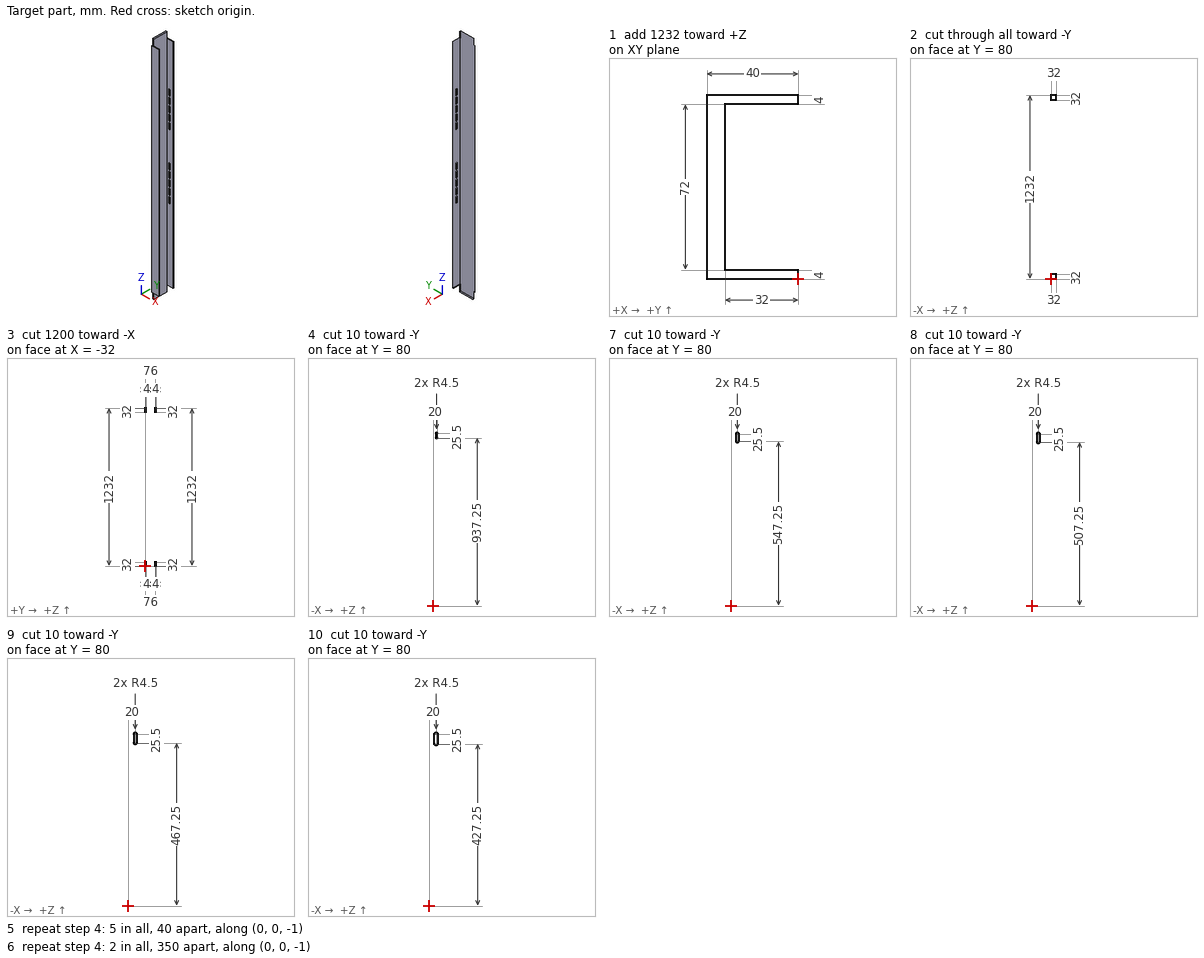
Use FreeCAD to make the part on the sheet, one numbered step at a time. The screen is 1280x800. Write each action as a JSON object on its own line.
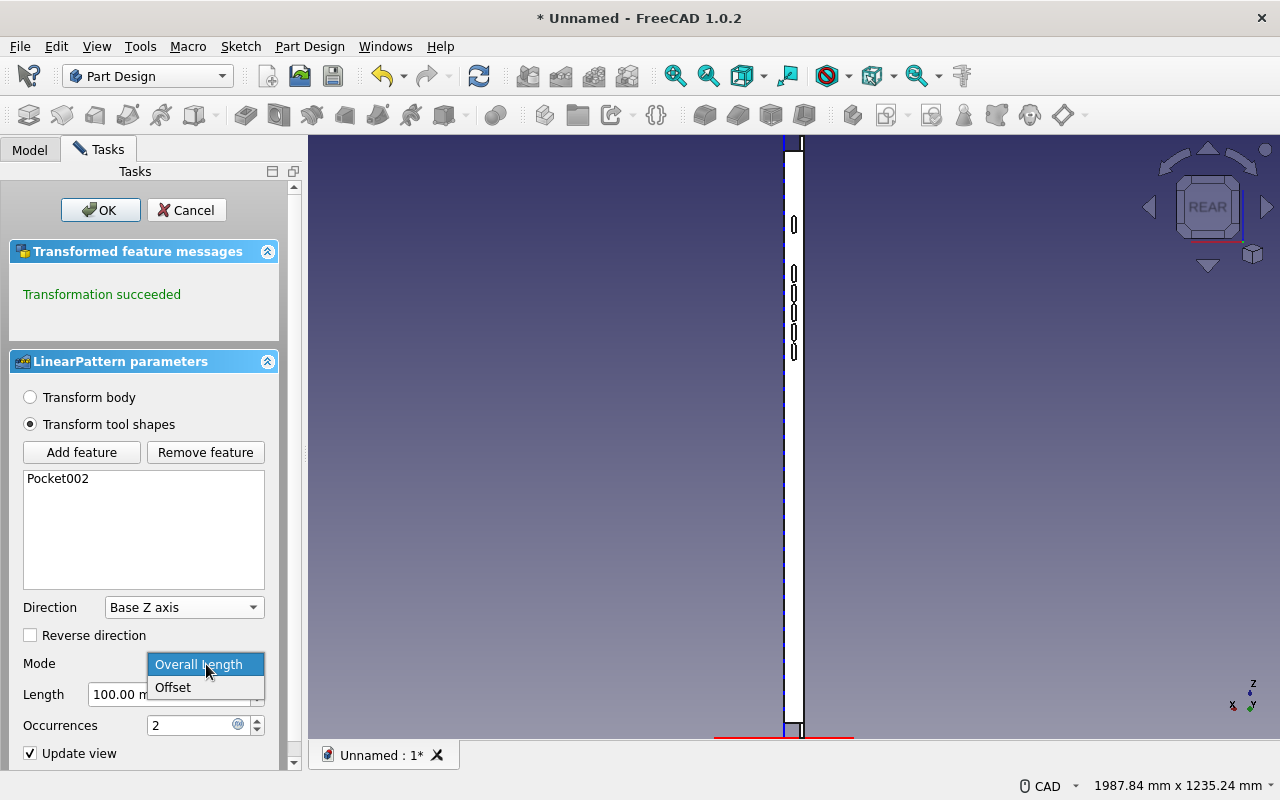
{"action": "left_click", "coordinate": [204, 688]}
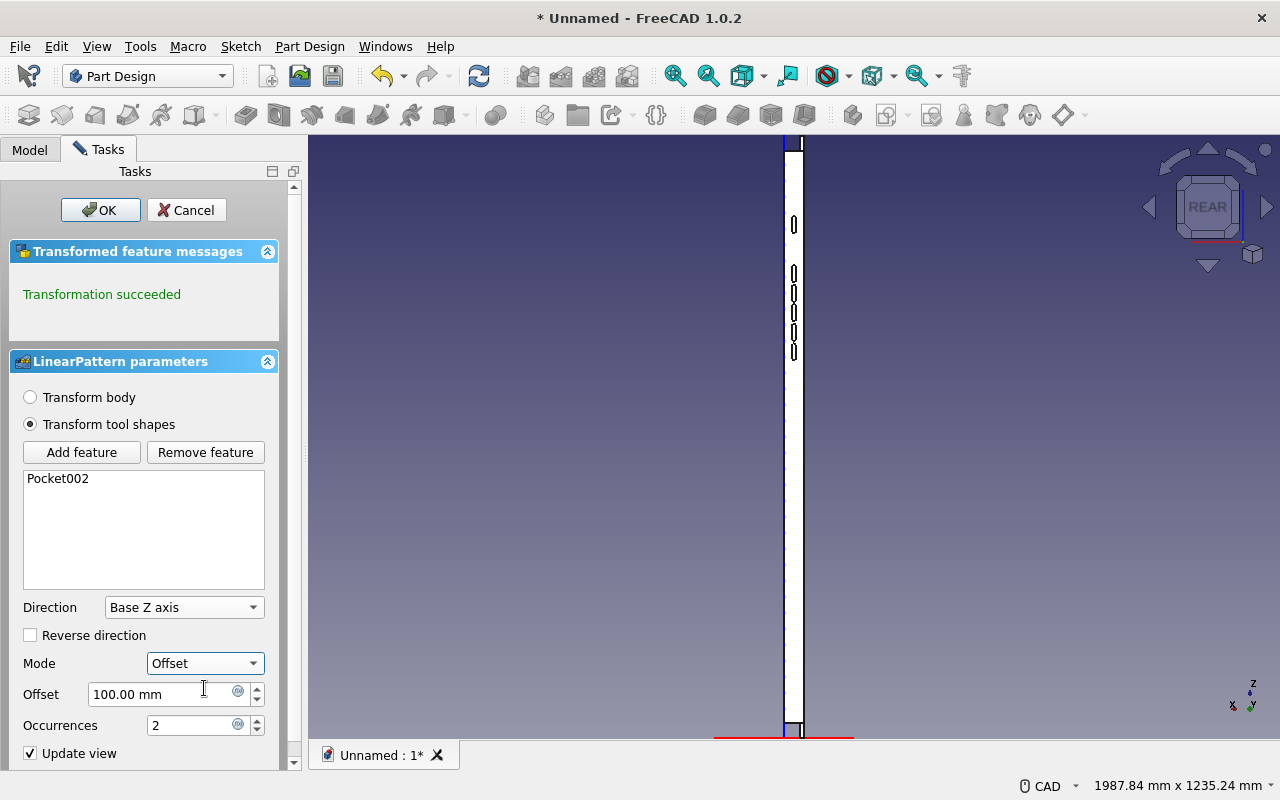
{"action": "triple_click", "coordinate": [170, 694]}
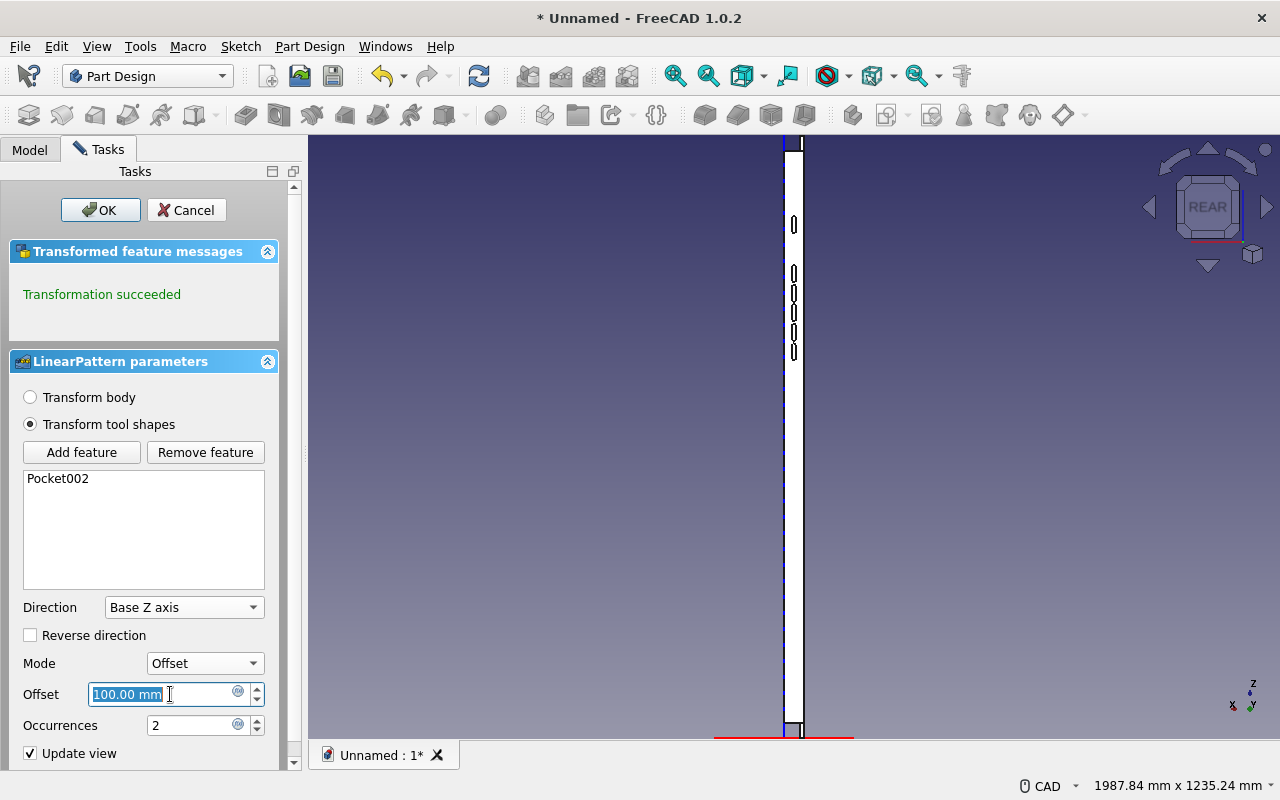
{"action": "type", "text": "350"}
{"action": "key", "text": "Tab"}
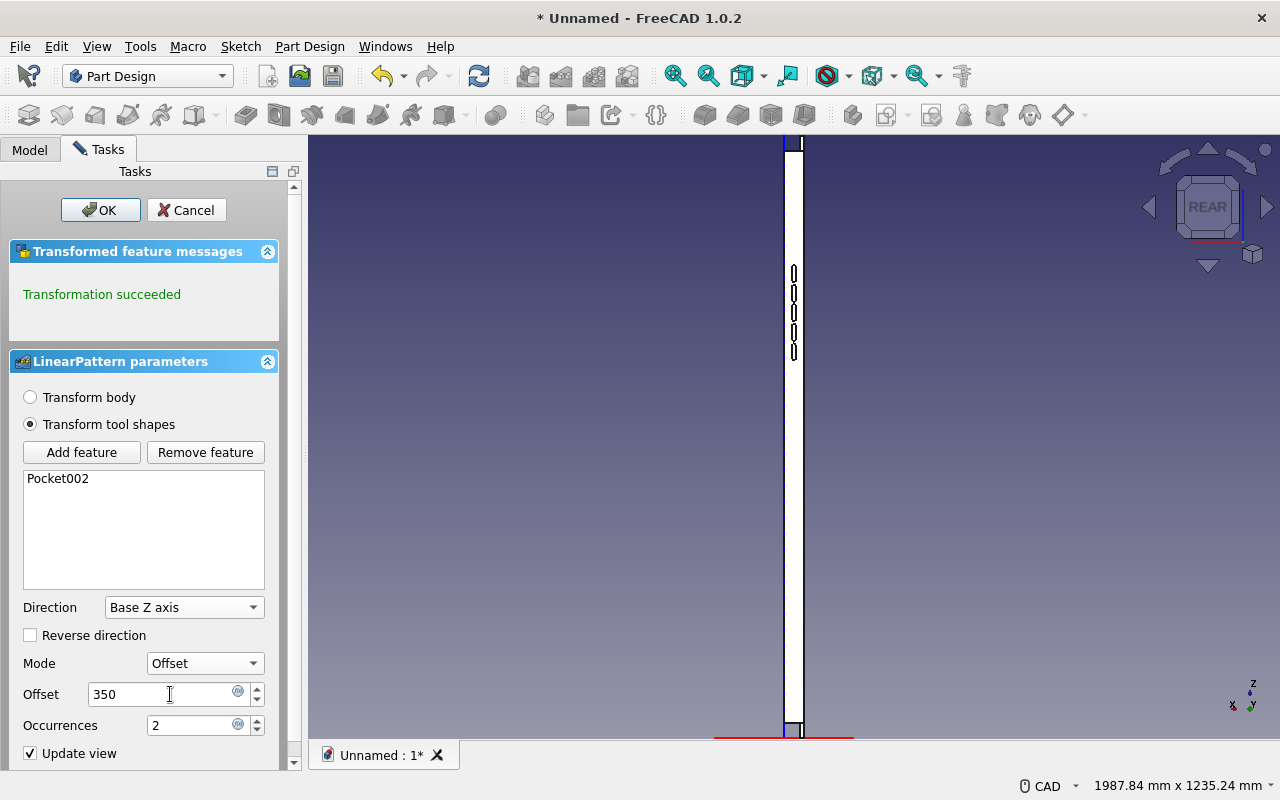
{"action": "triple_click", "coordinate": [199, 726]}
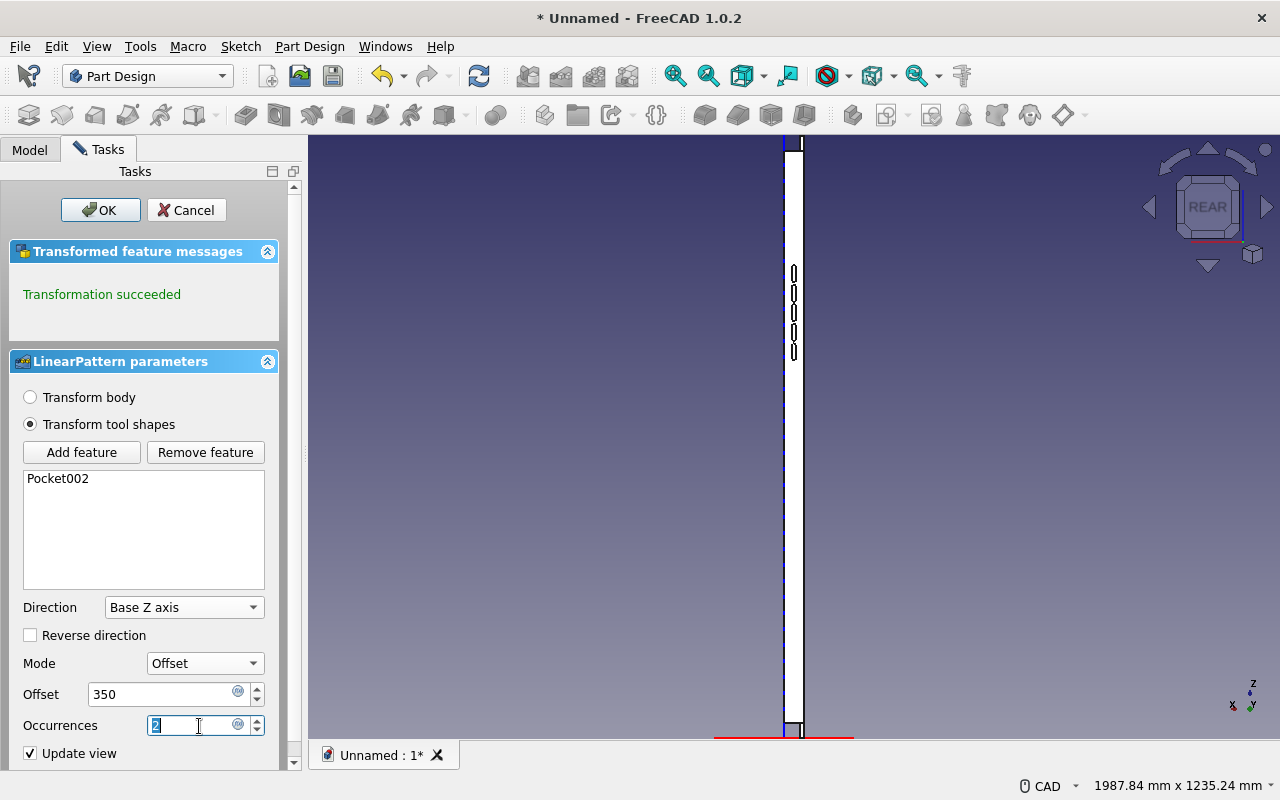
{"action": "type", "text": "2"}
{"action": "key", "text": "Tab"}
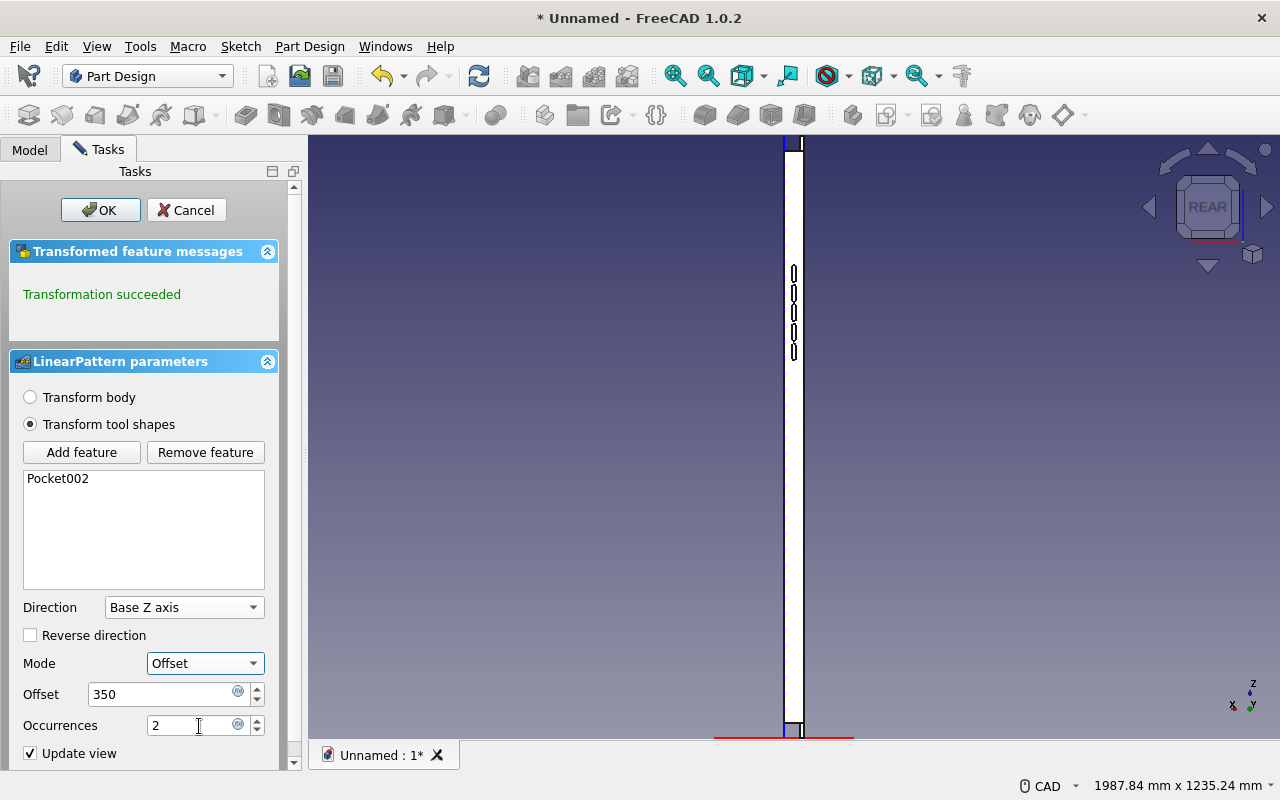
{"action": "left_click", "coordinate": [31, 635]}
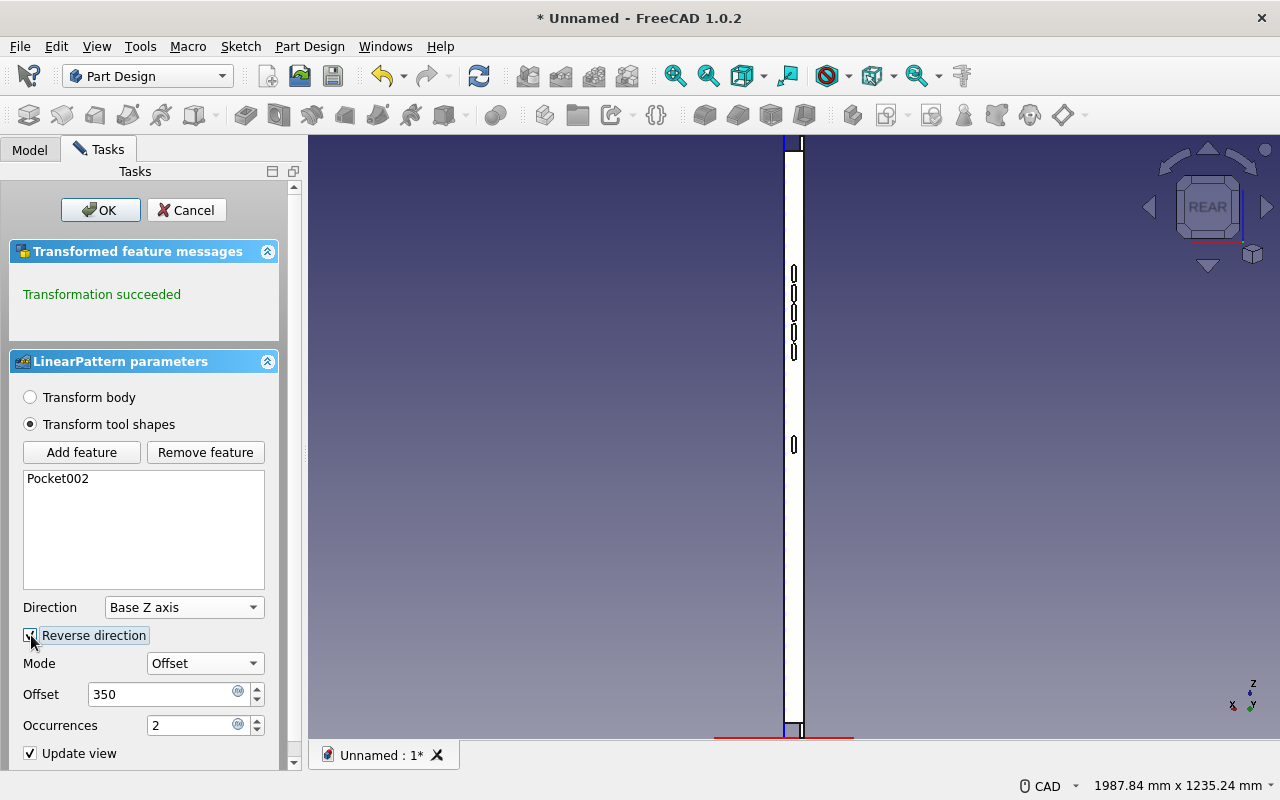
{"action": "left_click", "coordinate": [101, 210]}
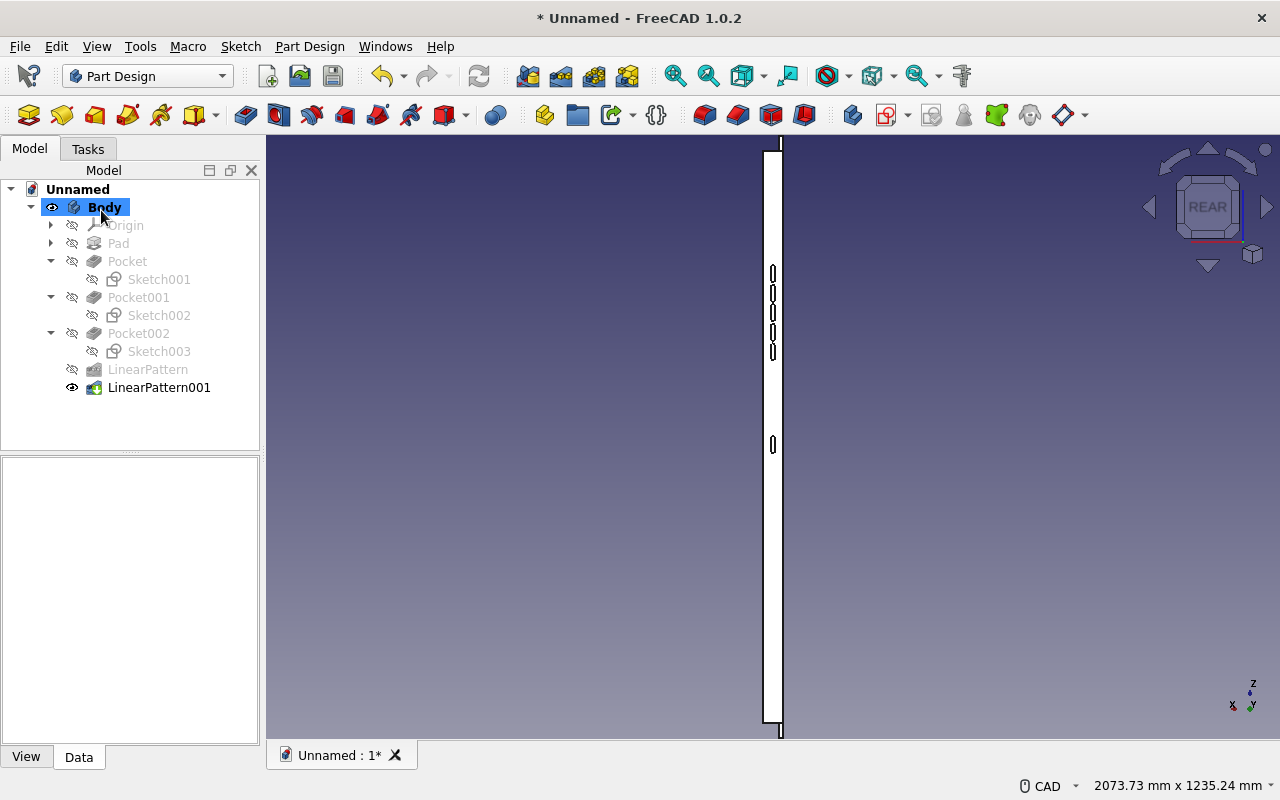
{"action": "left_click", "coordinate": [773, 191]}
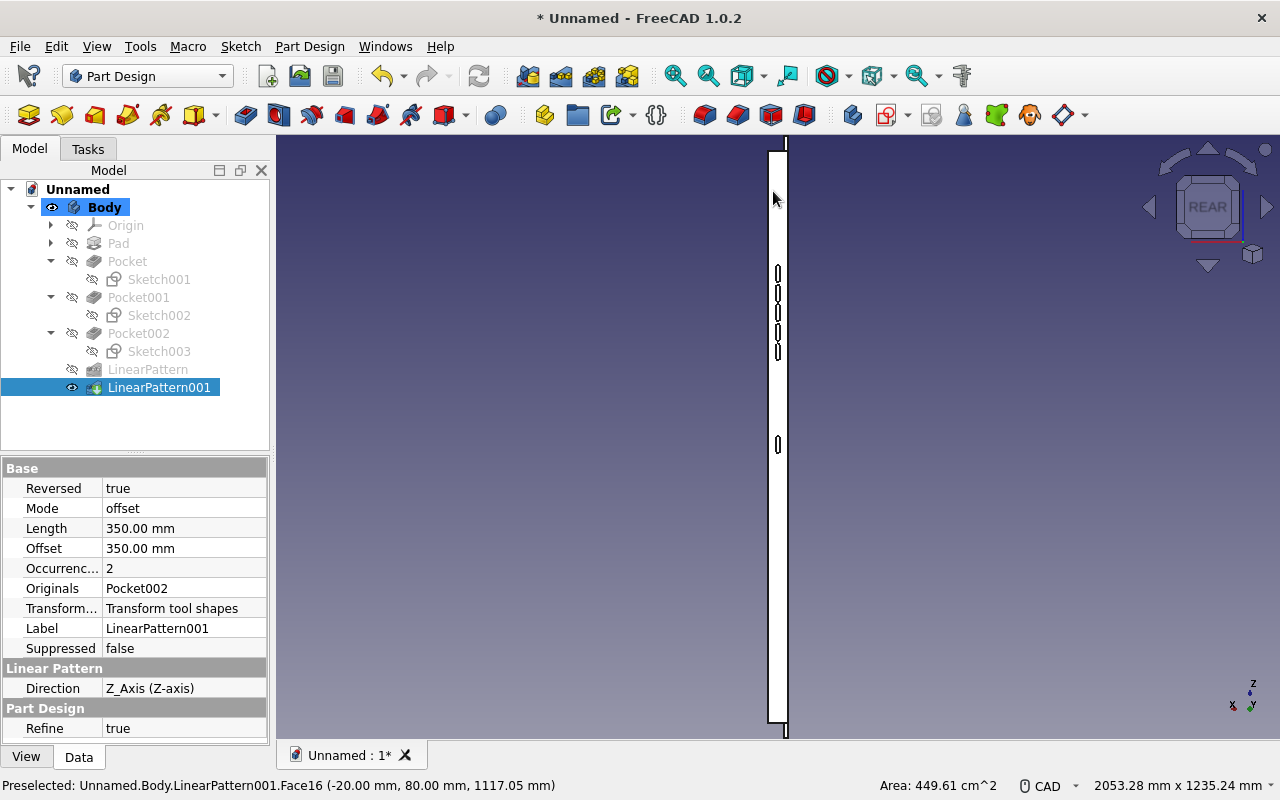
{"action": "left_click", "coordinate": [886, 116]}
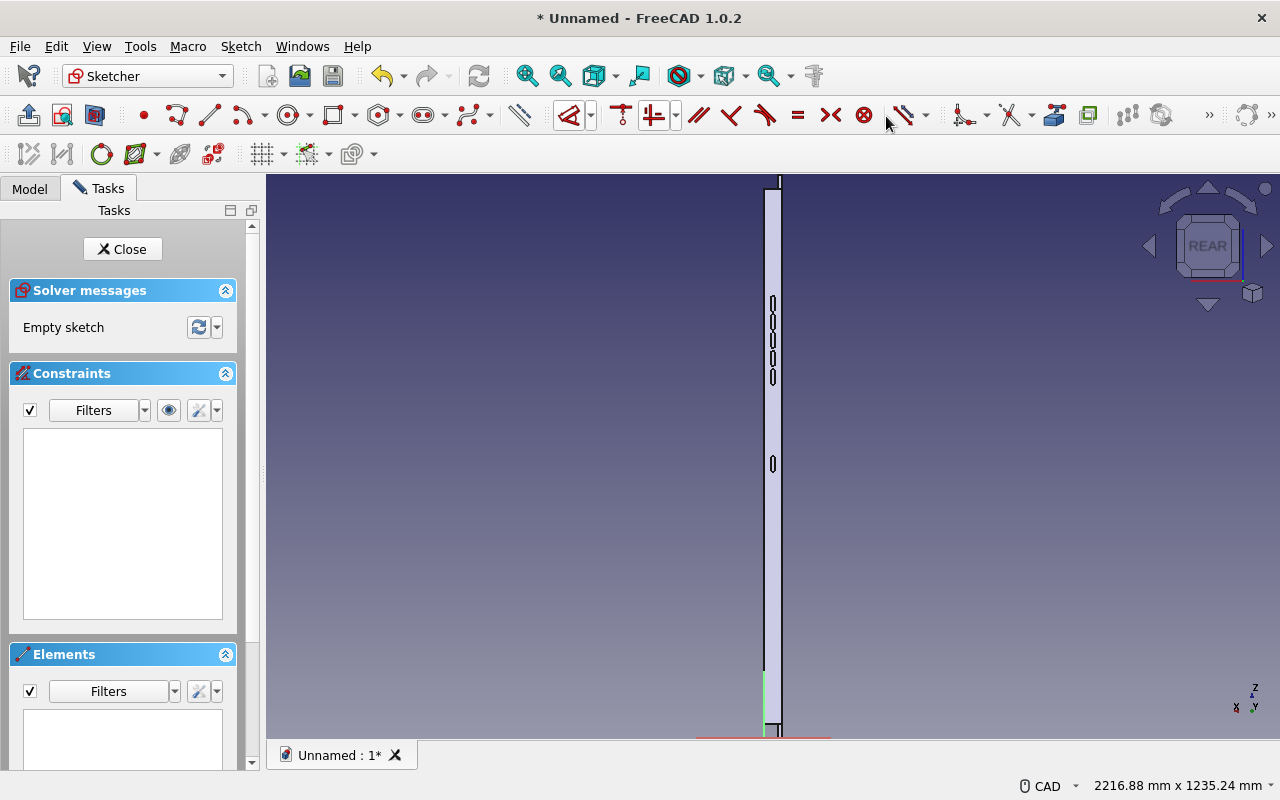
{"action": "scroll", "coordinate": [777, 483], "scroll_direction": "up", "scroll_amount": 15}